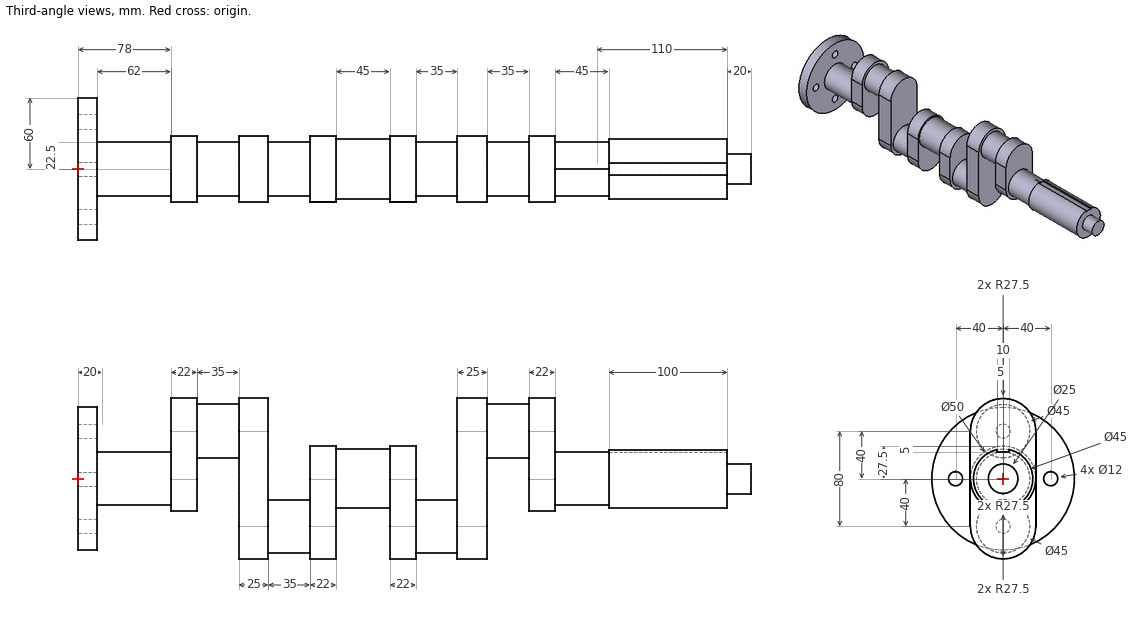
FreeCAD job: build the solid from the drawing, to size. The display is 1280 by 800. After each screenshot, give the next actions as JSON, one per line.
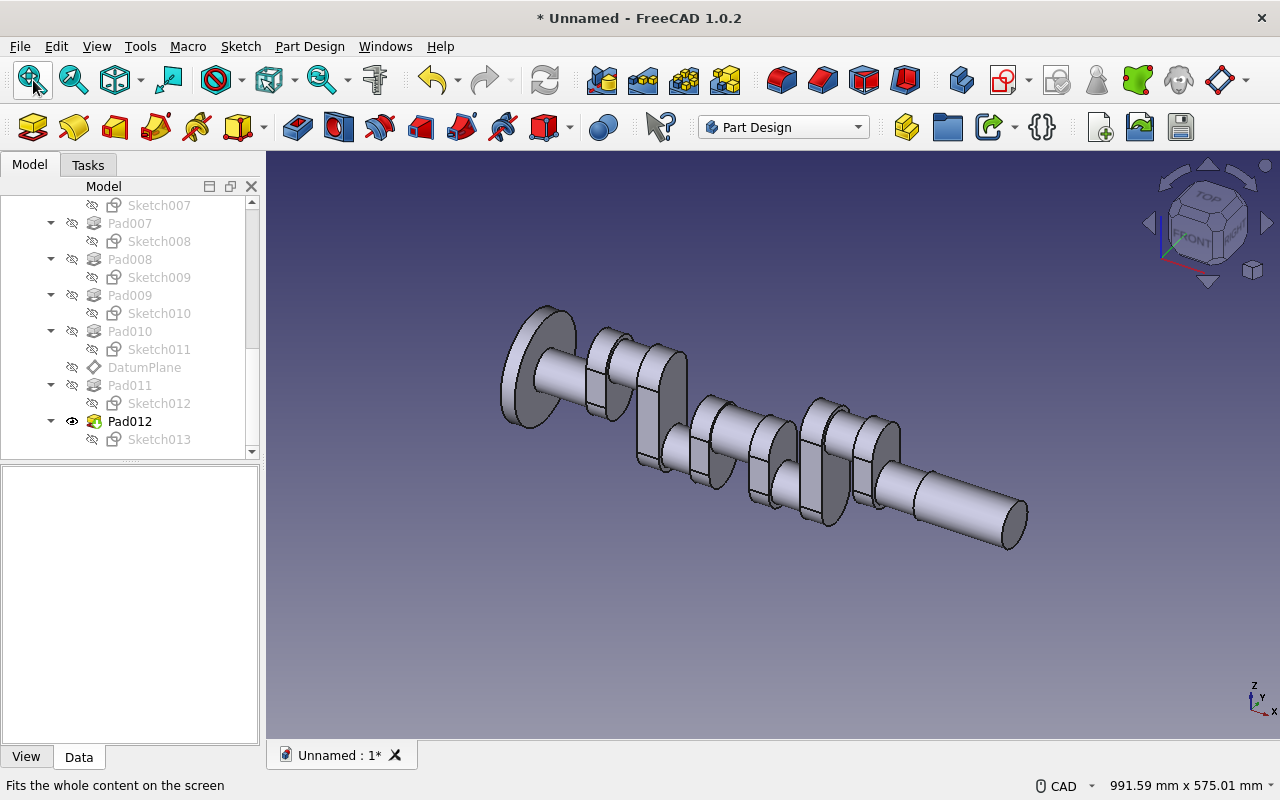
{"action": "left_click", "coordinate": [1015, 524]}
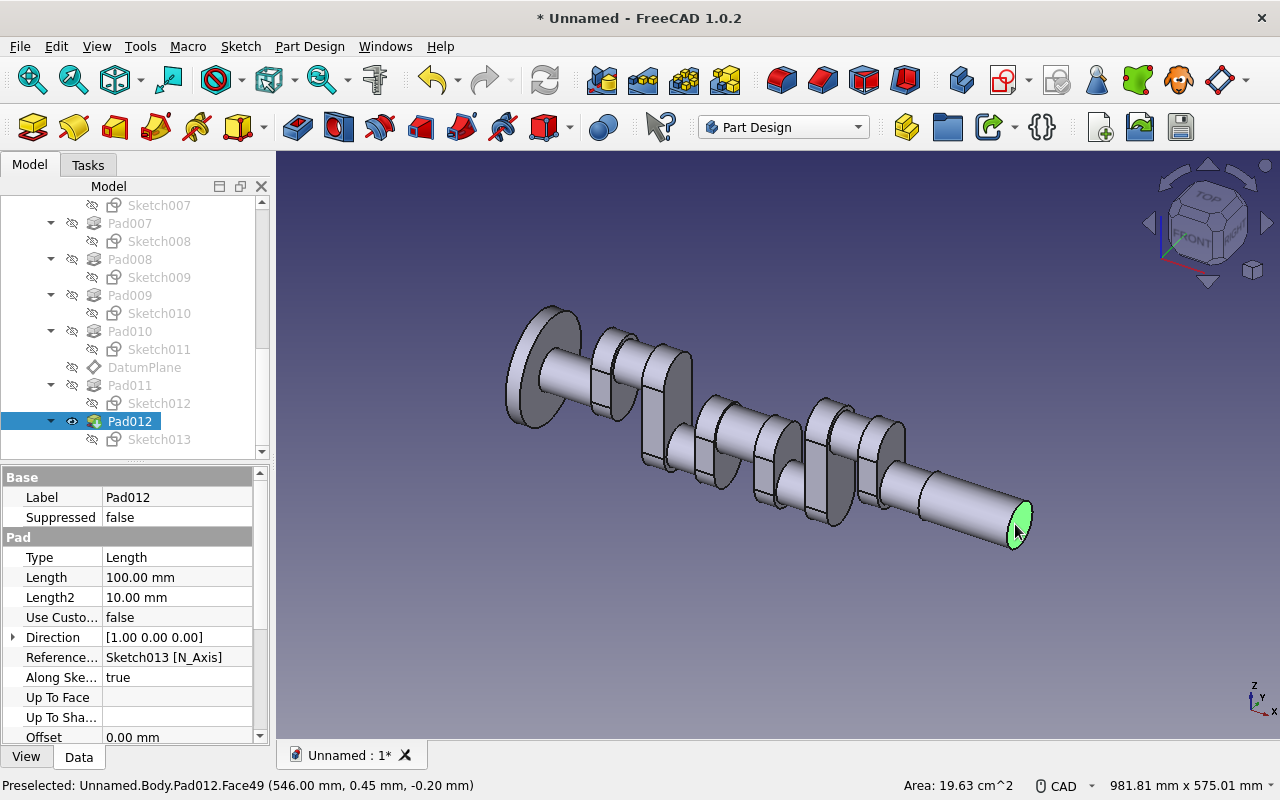
{"action": "left_click", "coordinate": [1002, 80]}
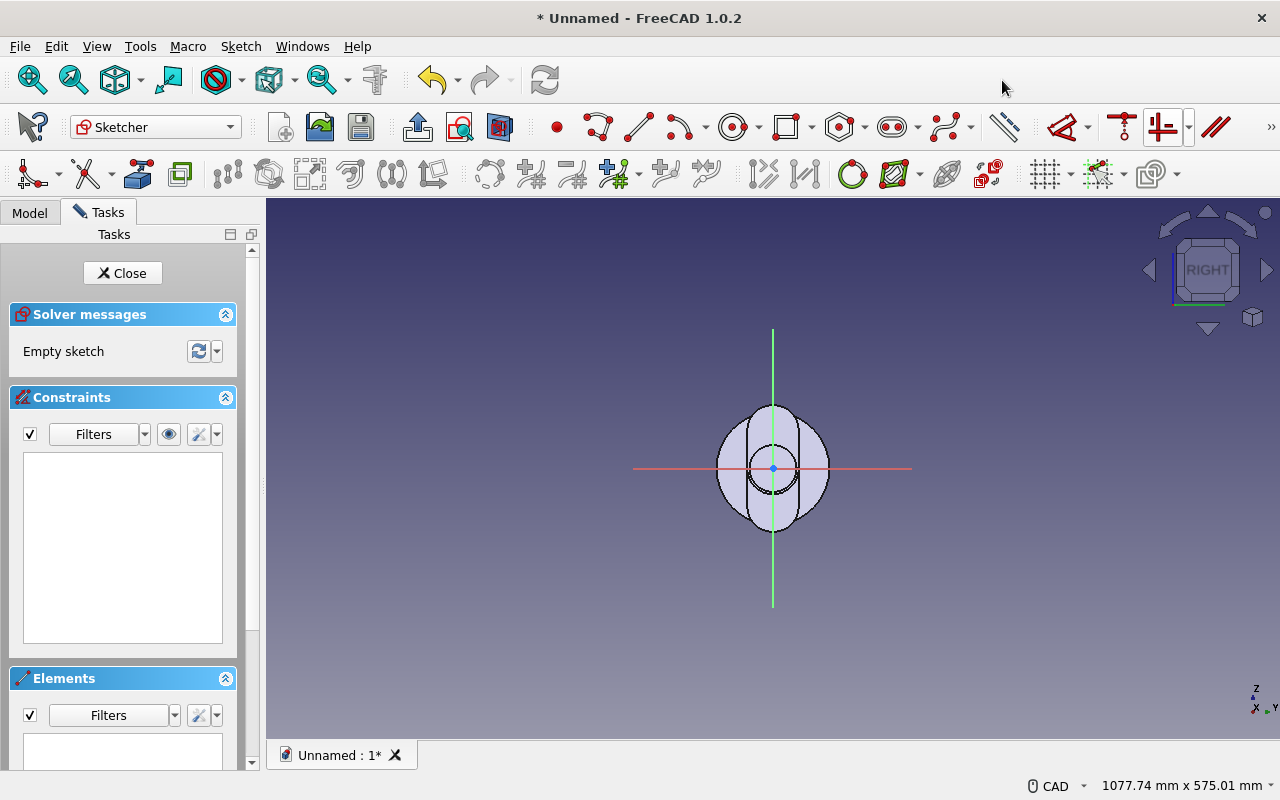
{"action": "scroll", "coordinate": [778, 468], "scroll_direction": "up", "scroll_amount": 13}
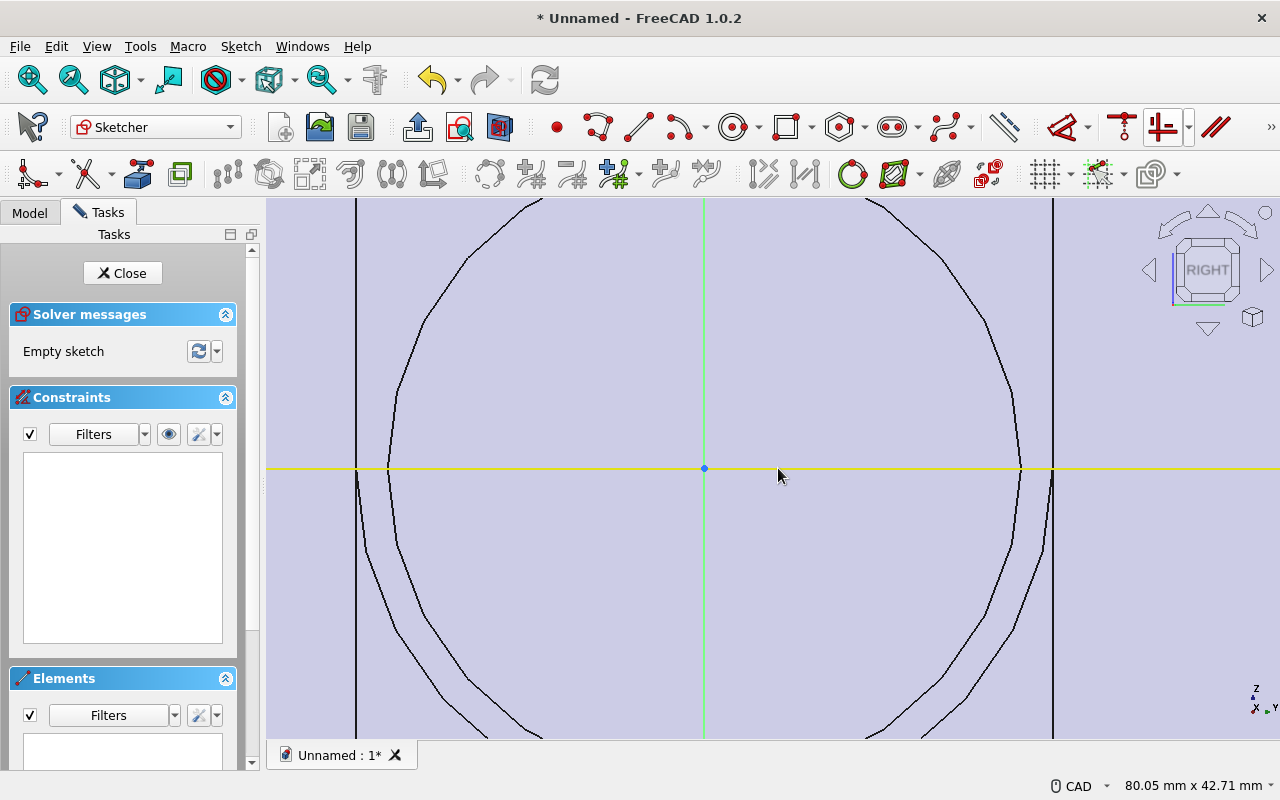
{"action": "left_click", "coordinate": [732, 128]}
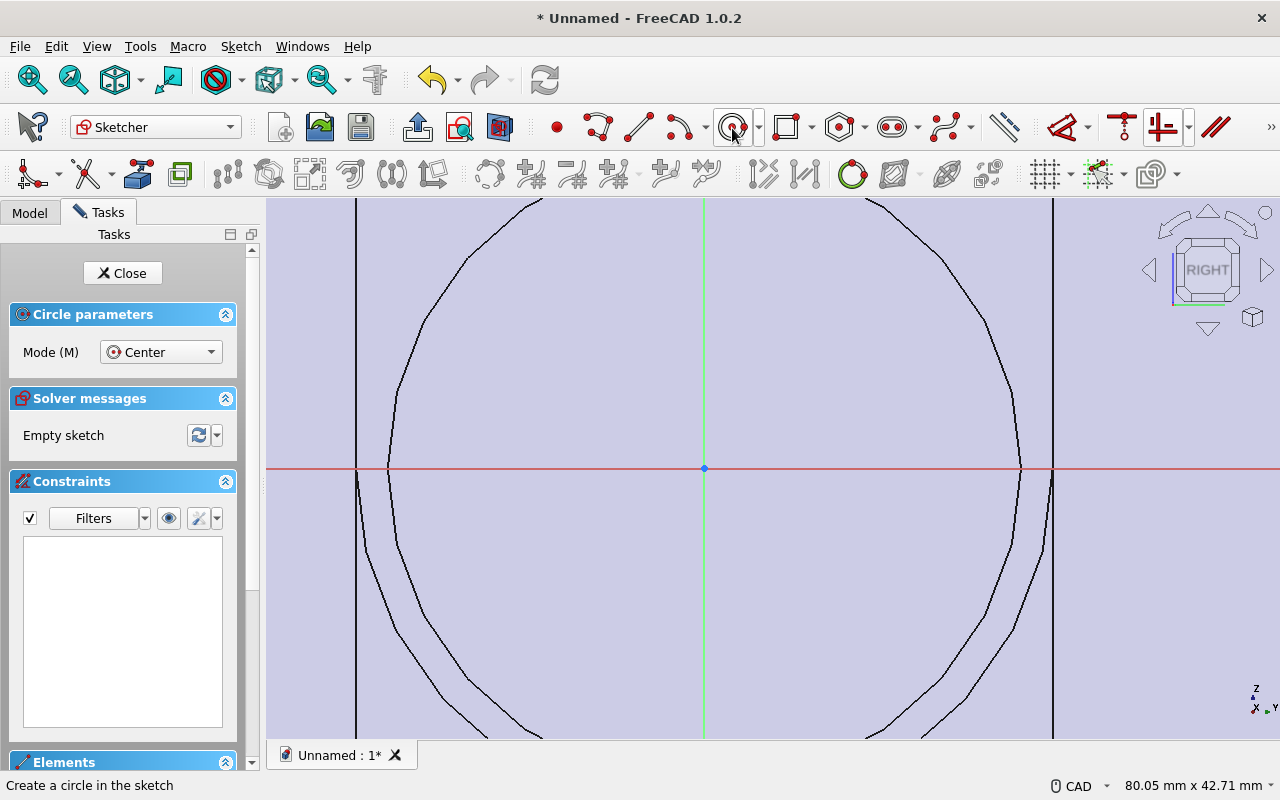
{"action": "left_click", "coordinate": [704, 468]}
{"action": "left_click", "coordinate": [816, 357]}
{"action": "key", "text": "Escape"}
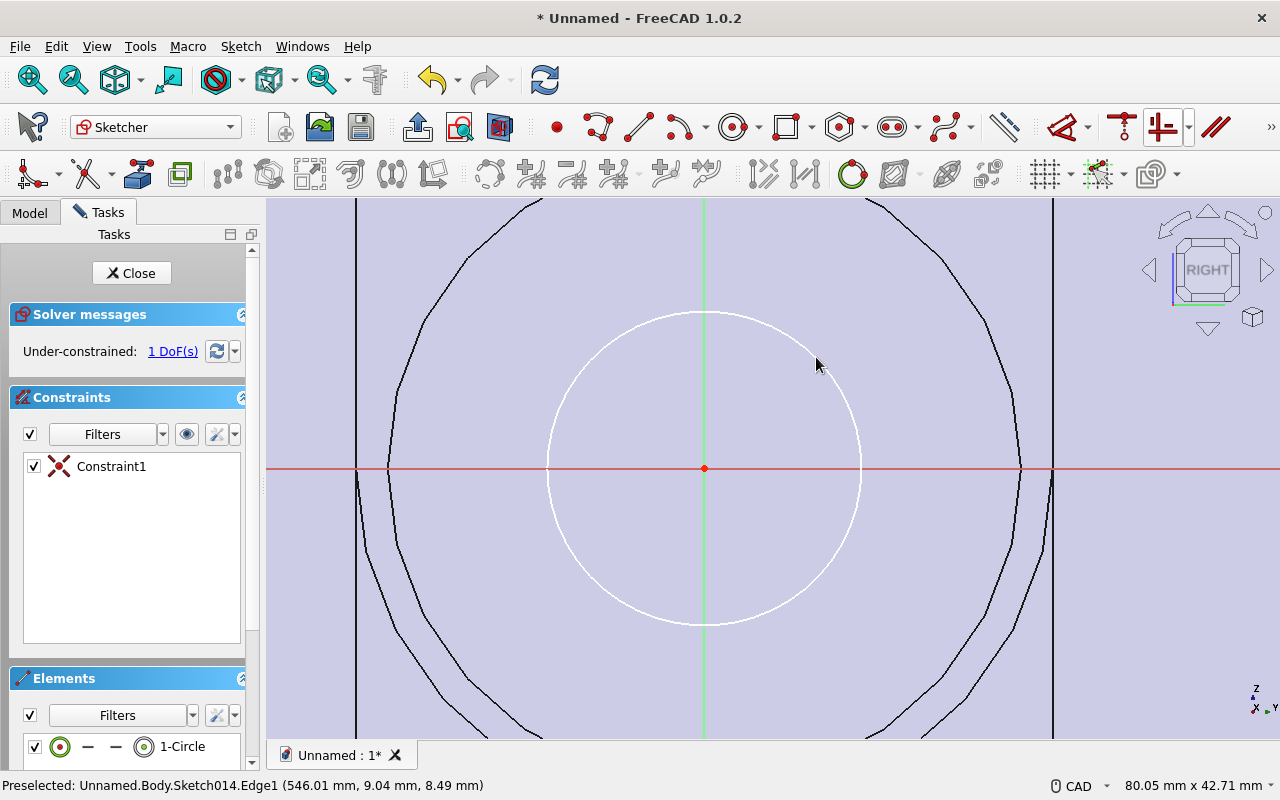
{"action": "left_click", "coordinate": [1062, 128]}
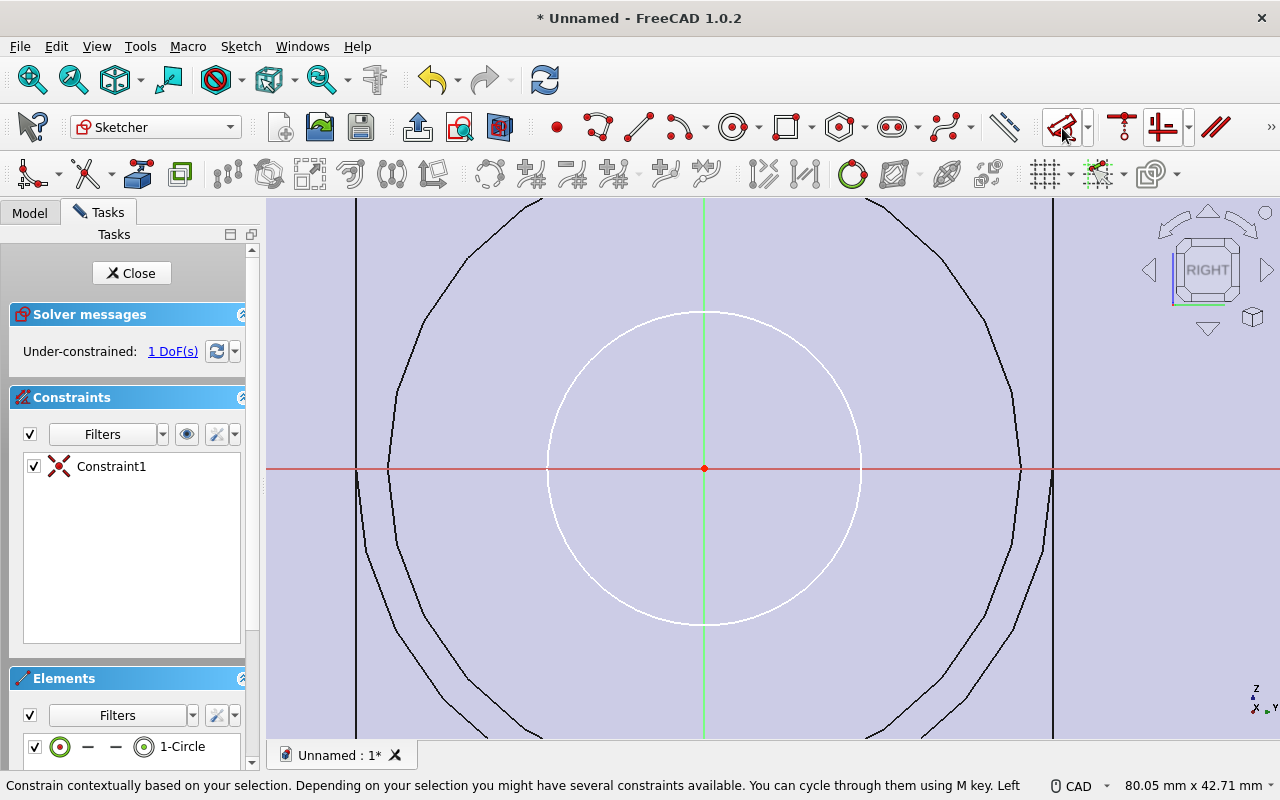
{"action": "left_click", "coordinate": [815, 357]}
{"action": "left_click", "coordinate": [838, 334]}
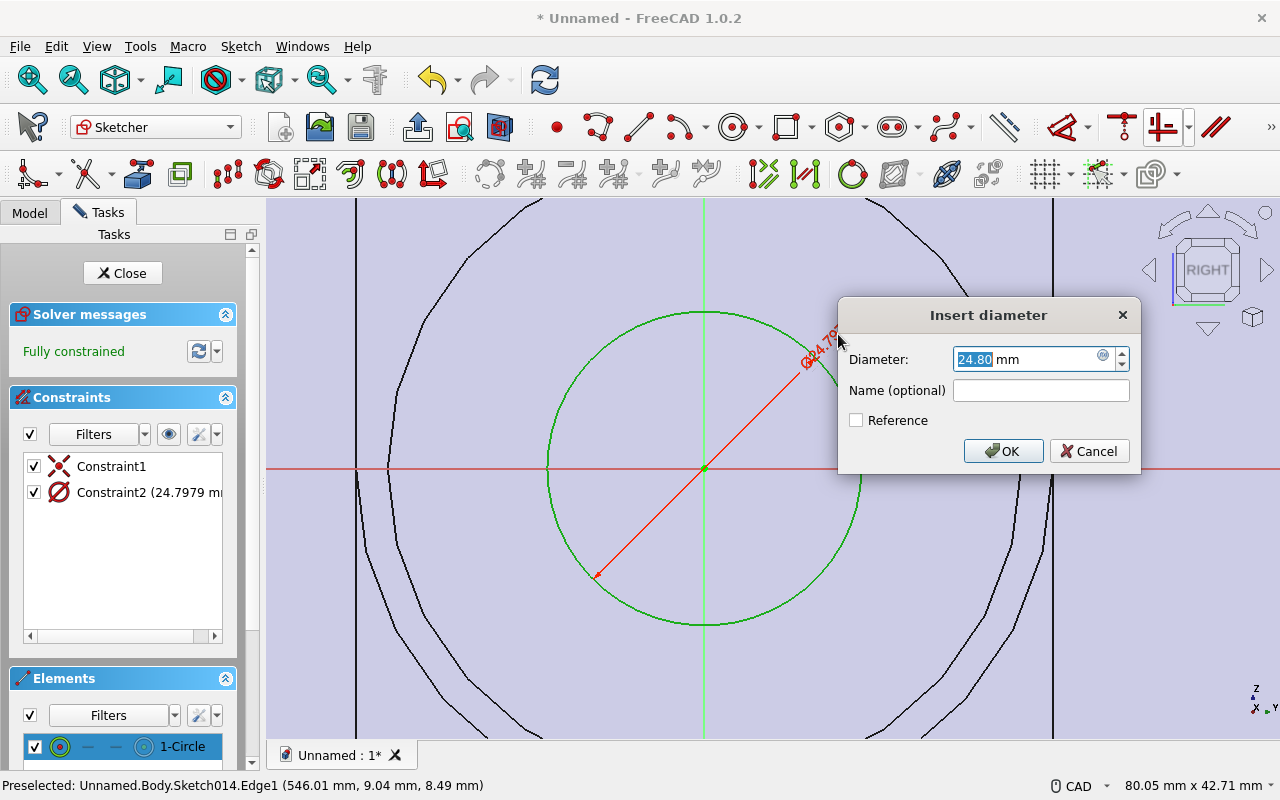
{"action": "type", "text": "25"}
{"action": "key", "text": "Return"}
{"action": "key", "text": "Escape"}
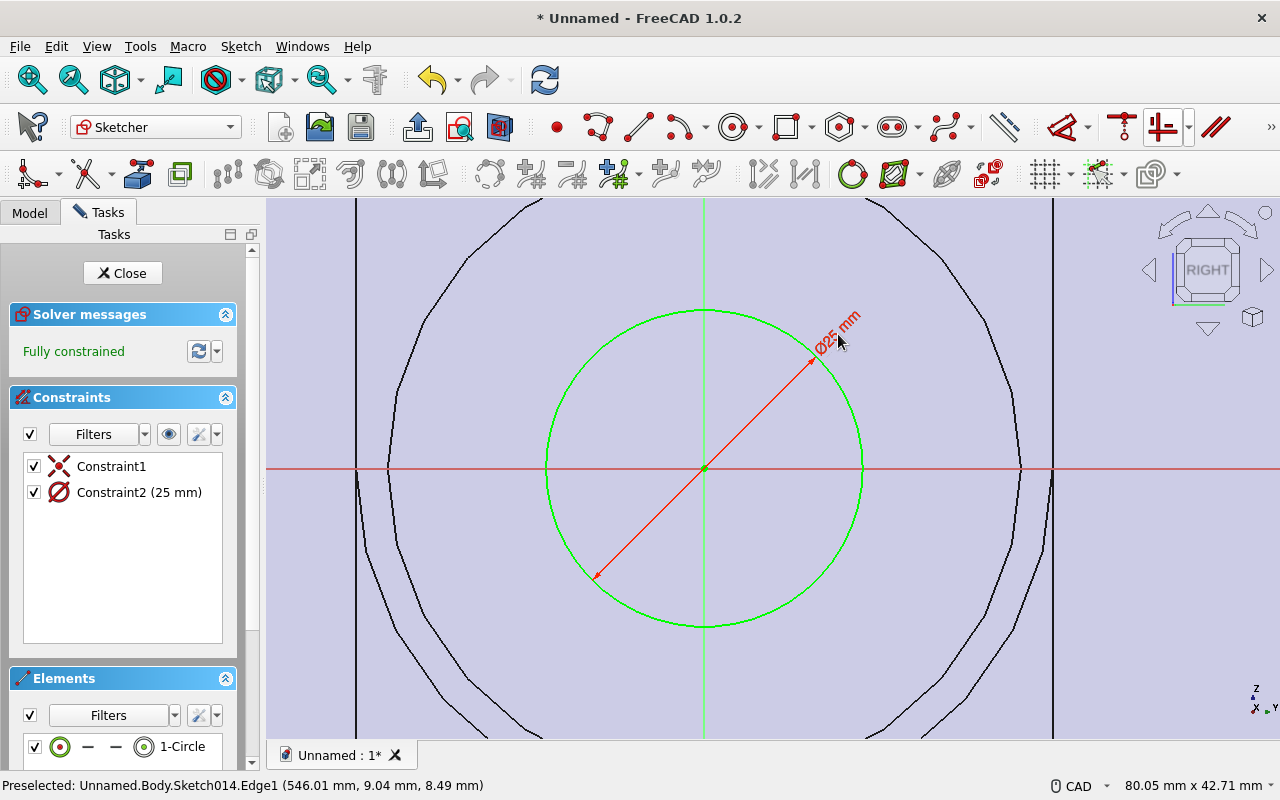
{"action": "left_click", "coordinate": [123, 273]}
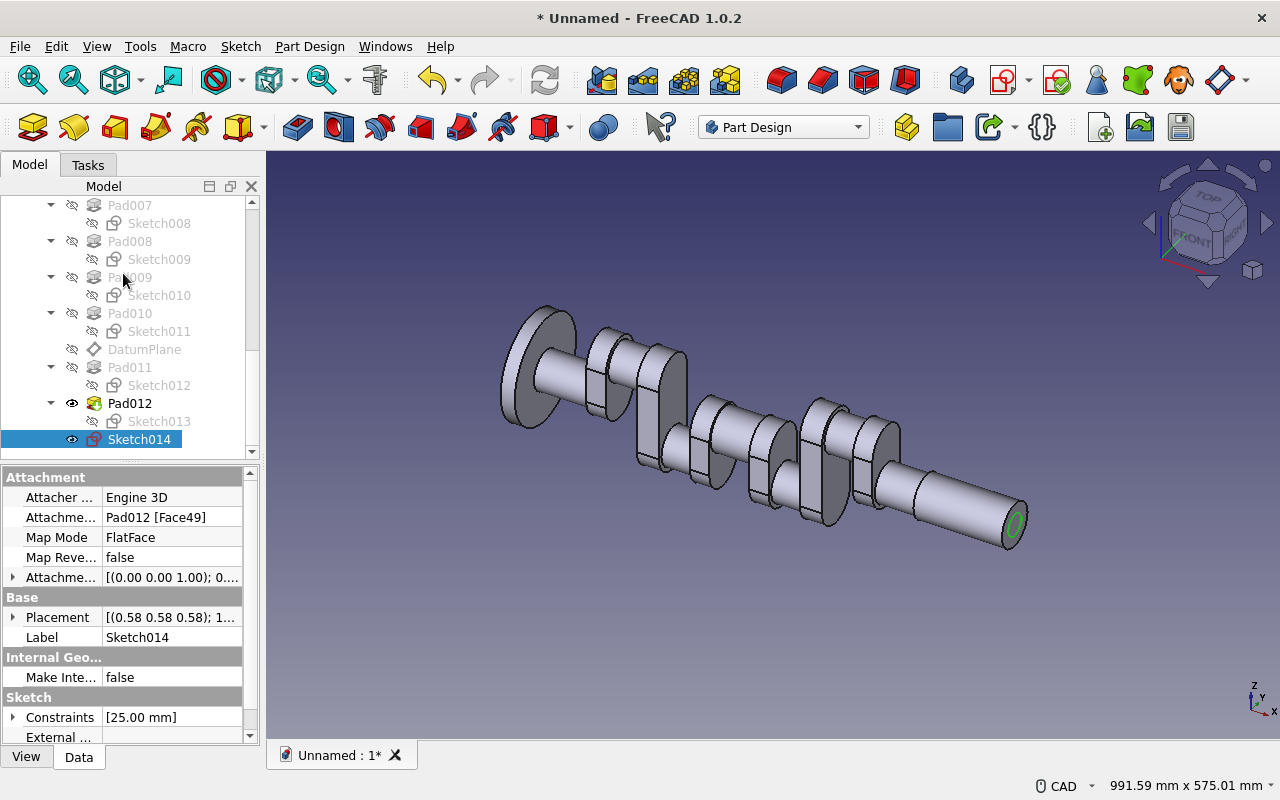
{"action": "left_click", "coordinate": [33, 128]}